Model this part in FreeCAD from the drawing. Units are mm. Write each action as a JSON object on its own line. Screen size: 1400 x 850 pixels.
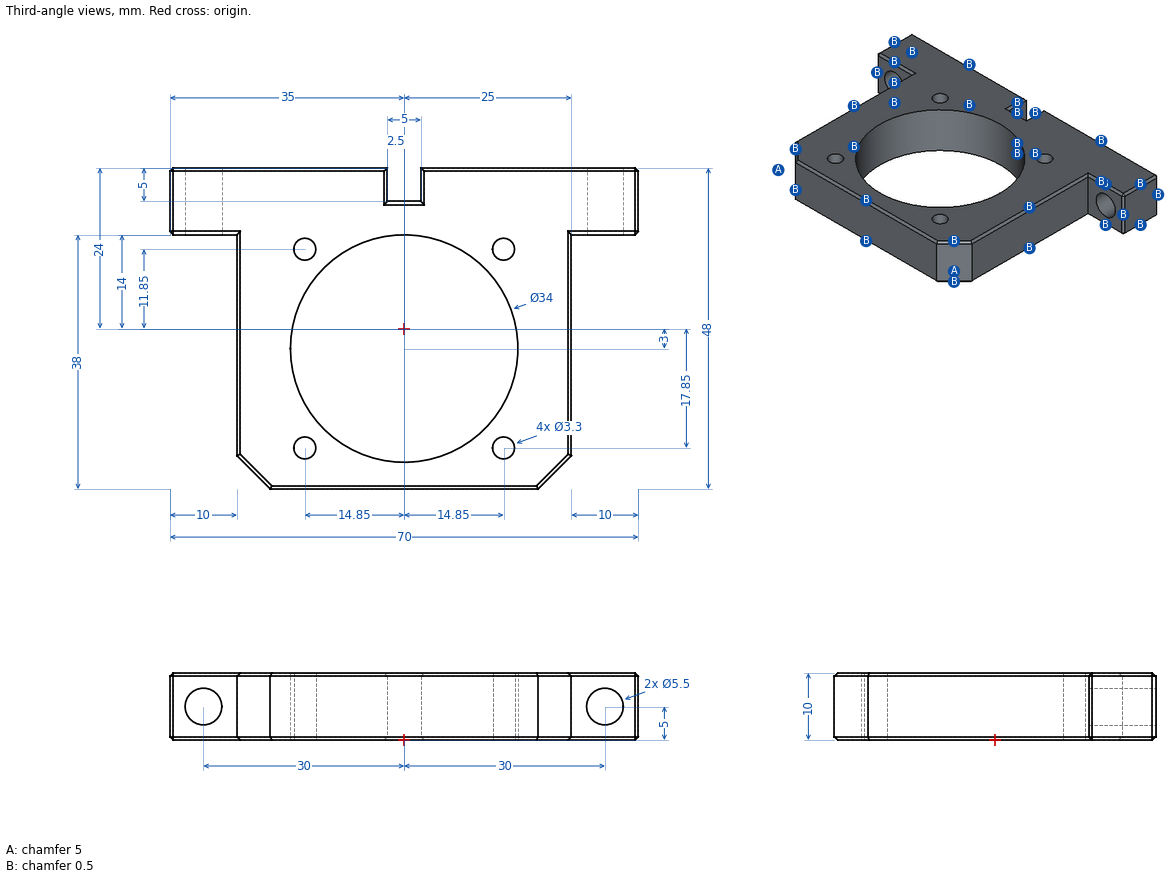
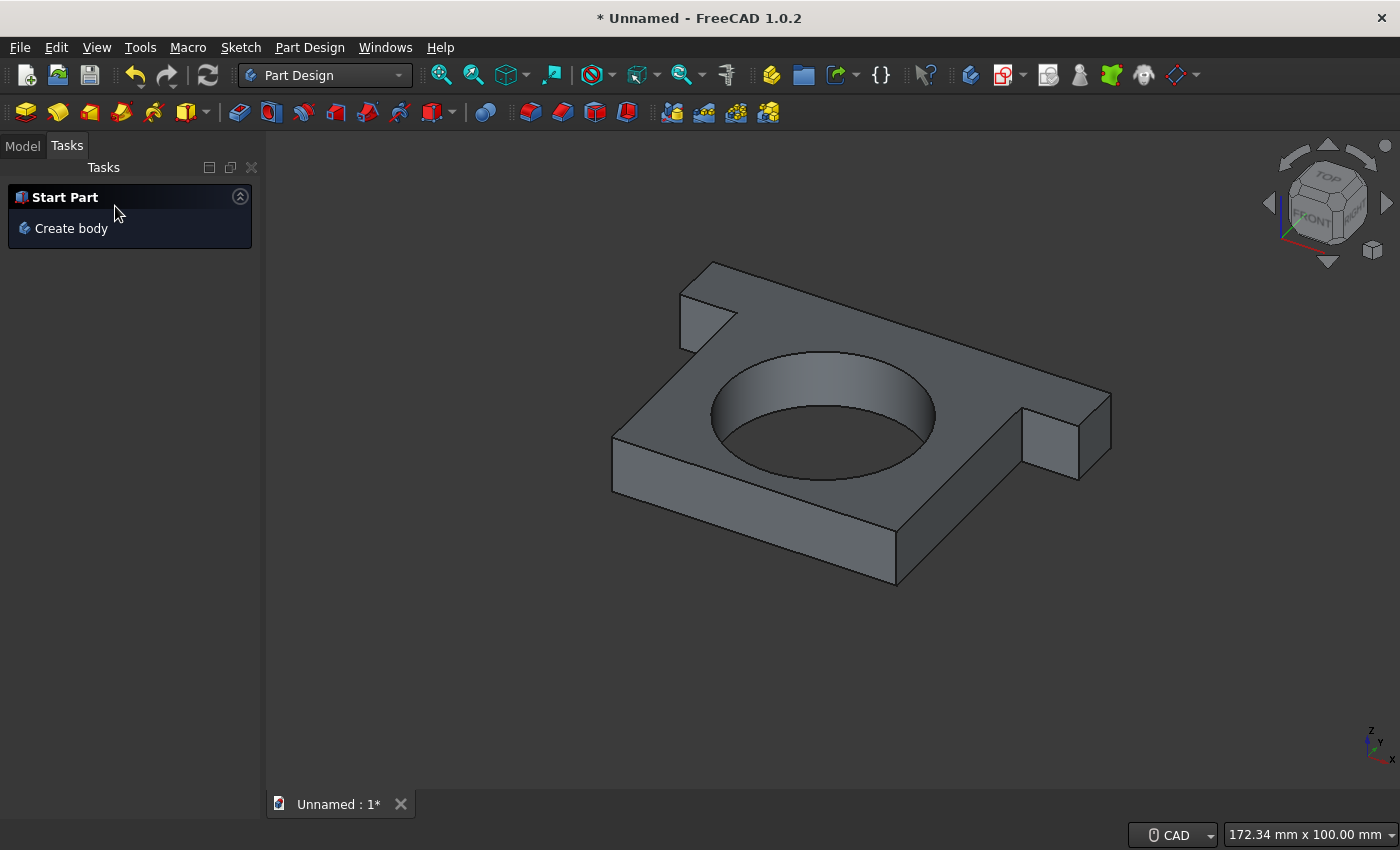
{"action": "left_click", "coordinate": [992, 398]}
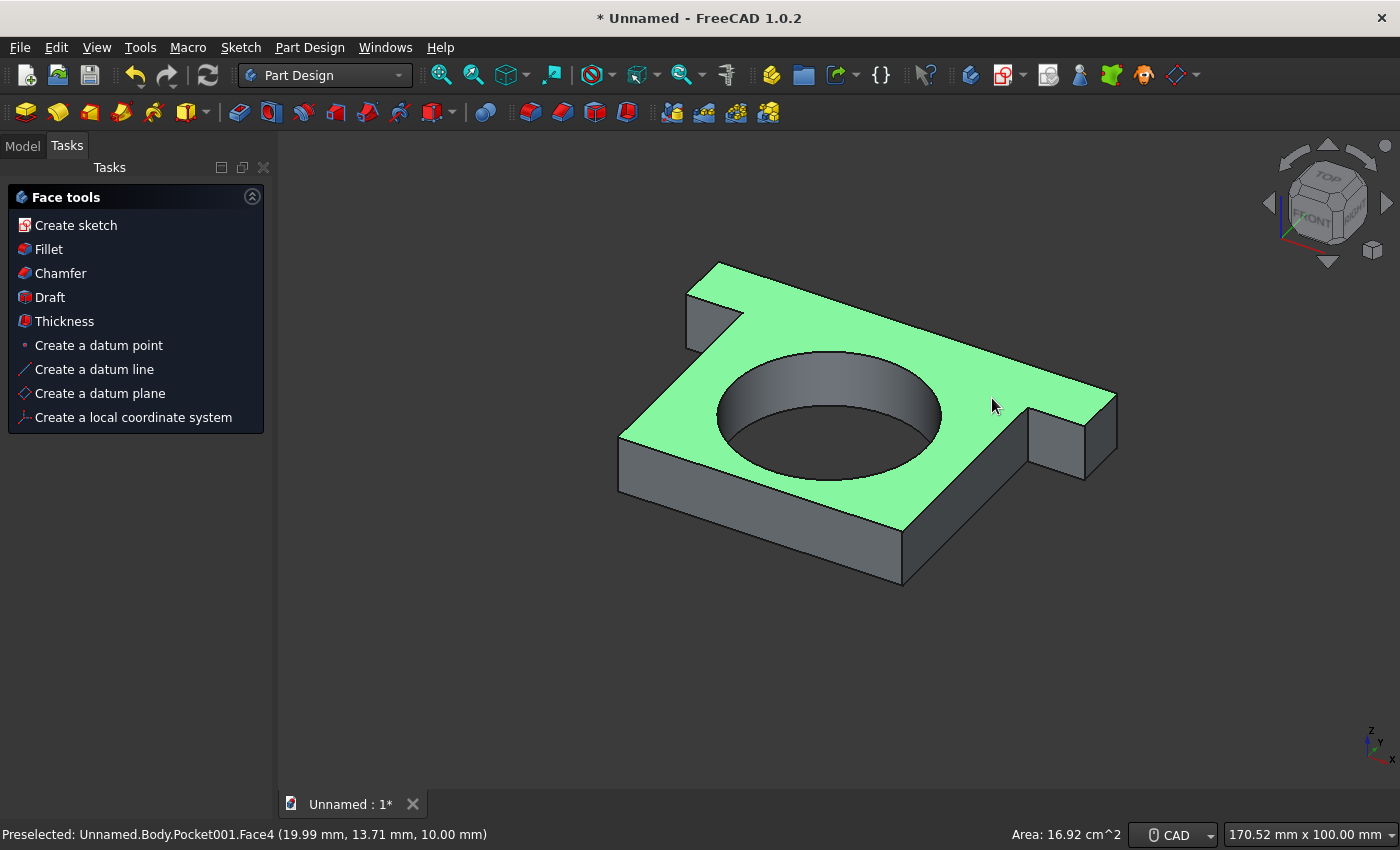
{"action": "left_click", "coordinate": [1004, 76]}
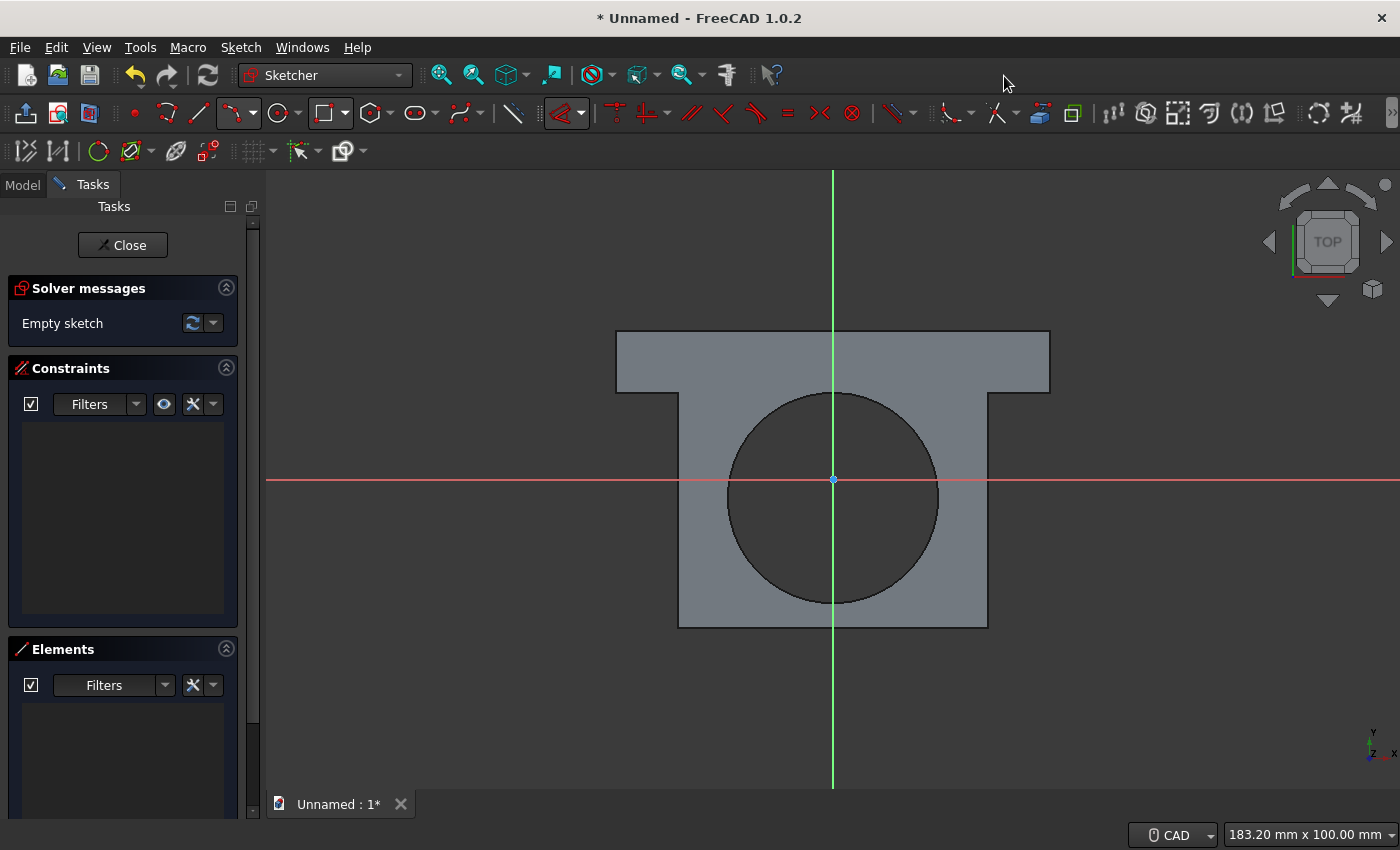
{"action": "scroll", "coordinate": [916, 521], "scroll_direction": "up", "scroll_amount": 3}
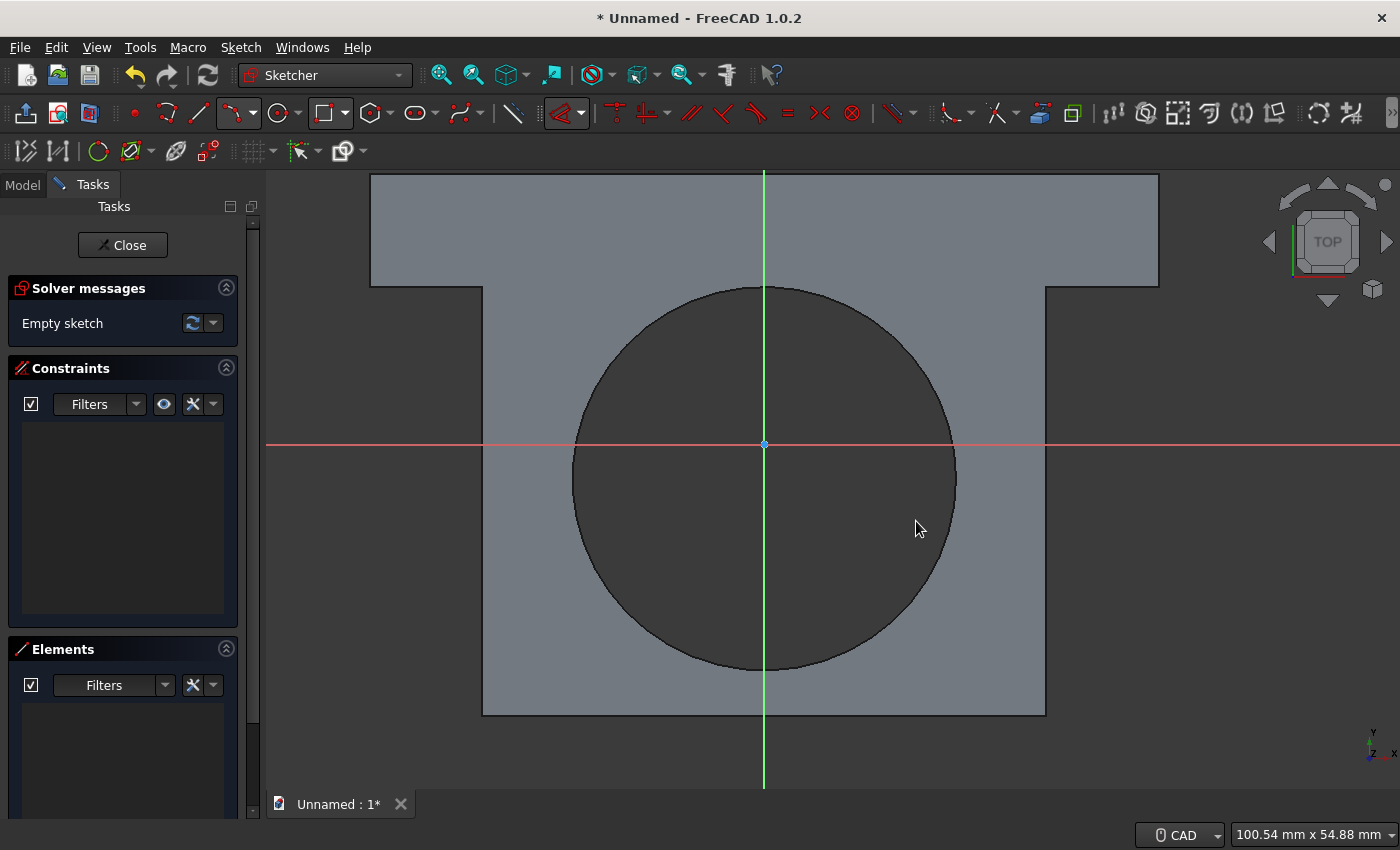
{"action": "key", "text": "g c"}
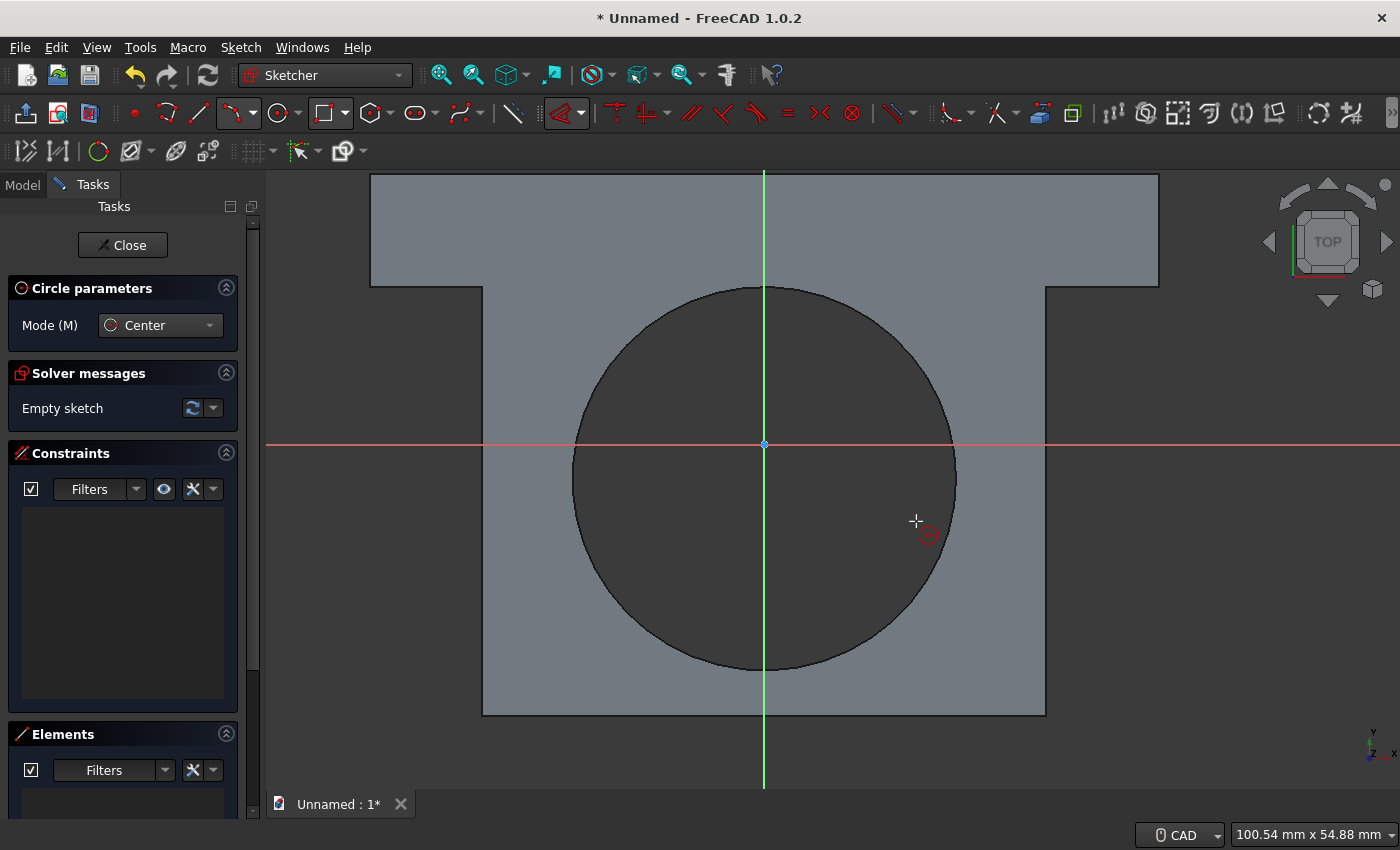
{"action": "left_click", "coordinate": [932, 646]}
{"action": "left_click", "coordinate": [945, 633]}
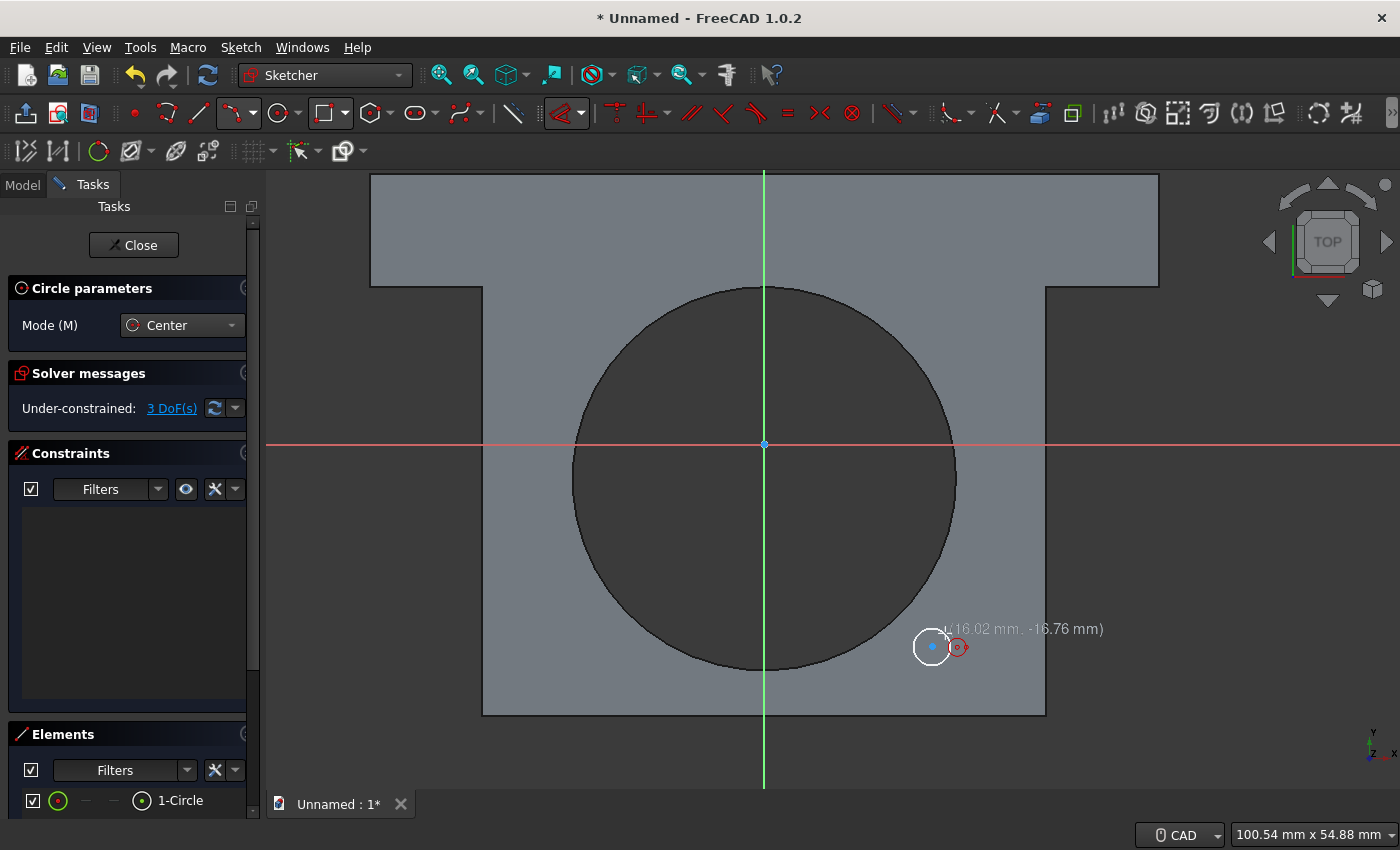
{"action": "left_click", "coordinate": [597, 646]}
{"action": "left_click", "coordinate": [610, 633]}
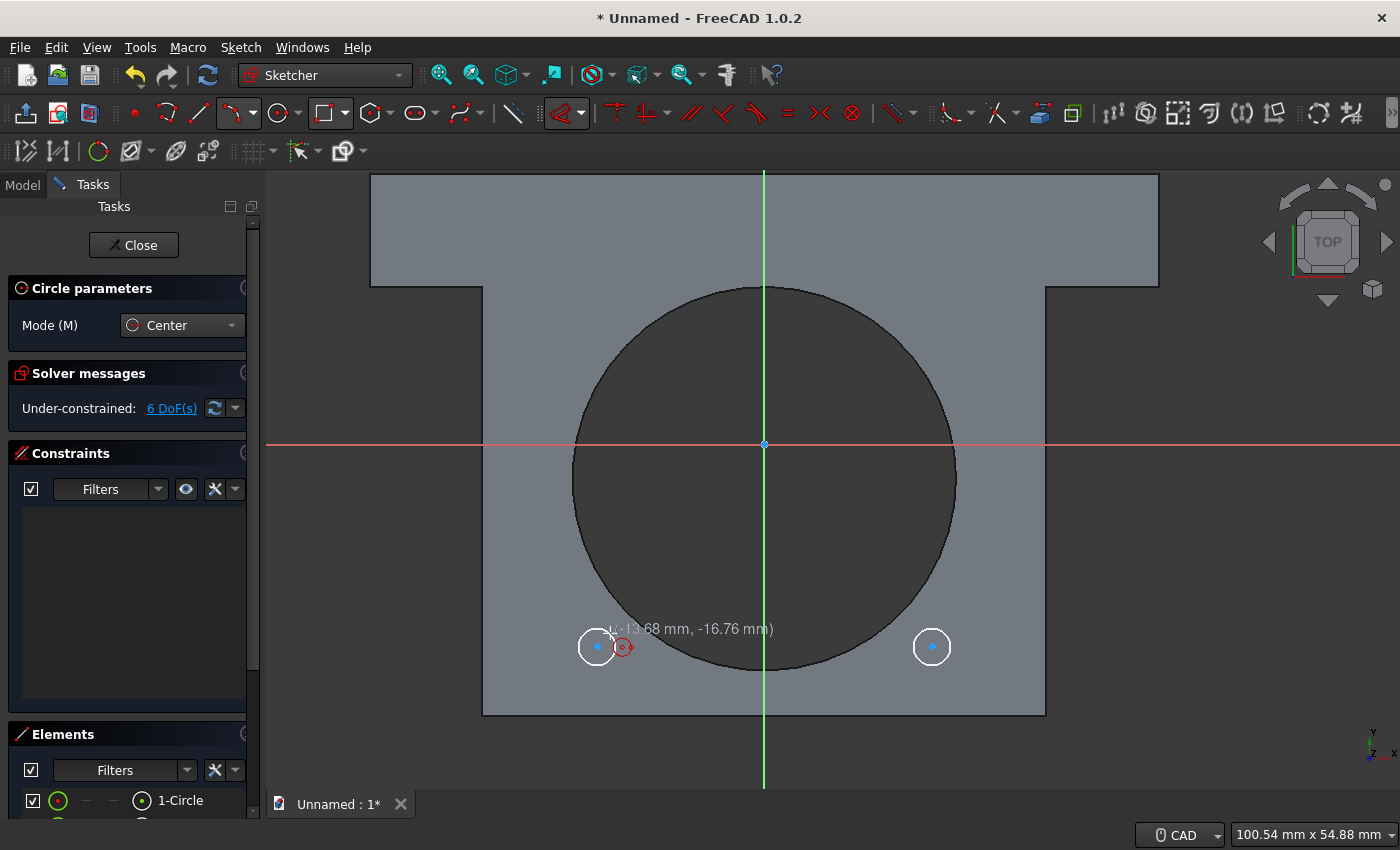
{"action": "left_click", "coordinate": [597, 311]}
{"action": "left_click", "coordinate": [610, 298]}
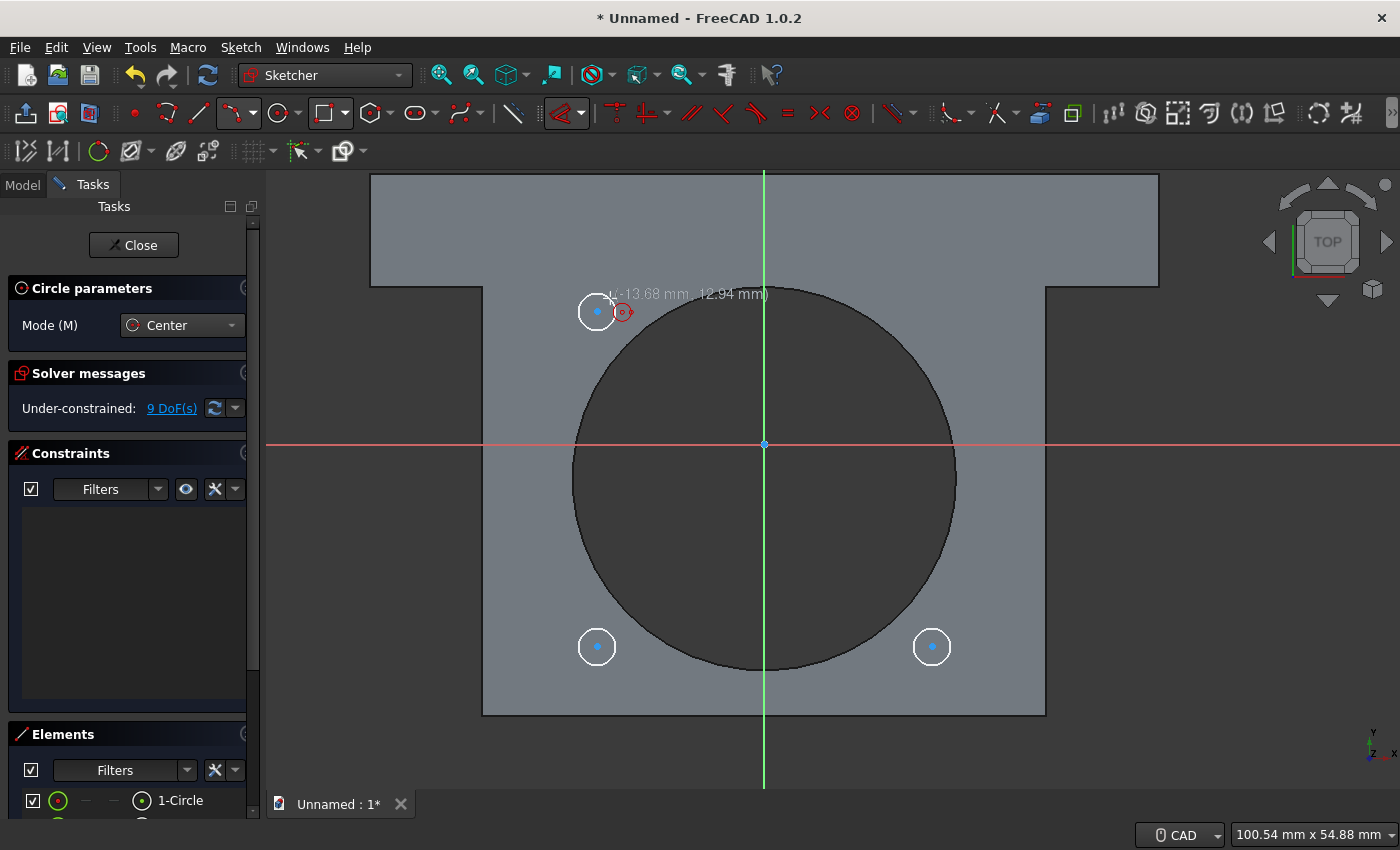
{"action": "left_click", "coordinate": [932, 311]}
{"action": "left_click", "coordinate": [945, 298]}
{"action": "key", "text": "Escape"}